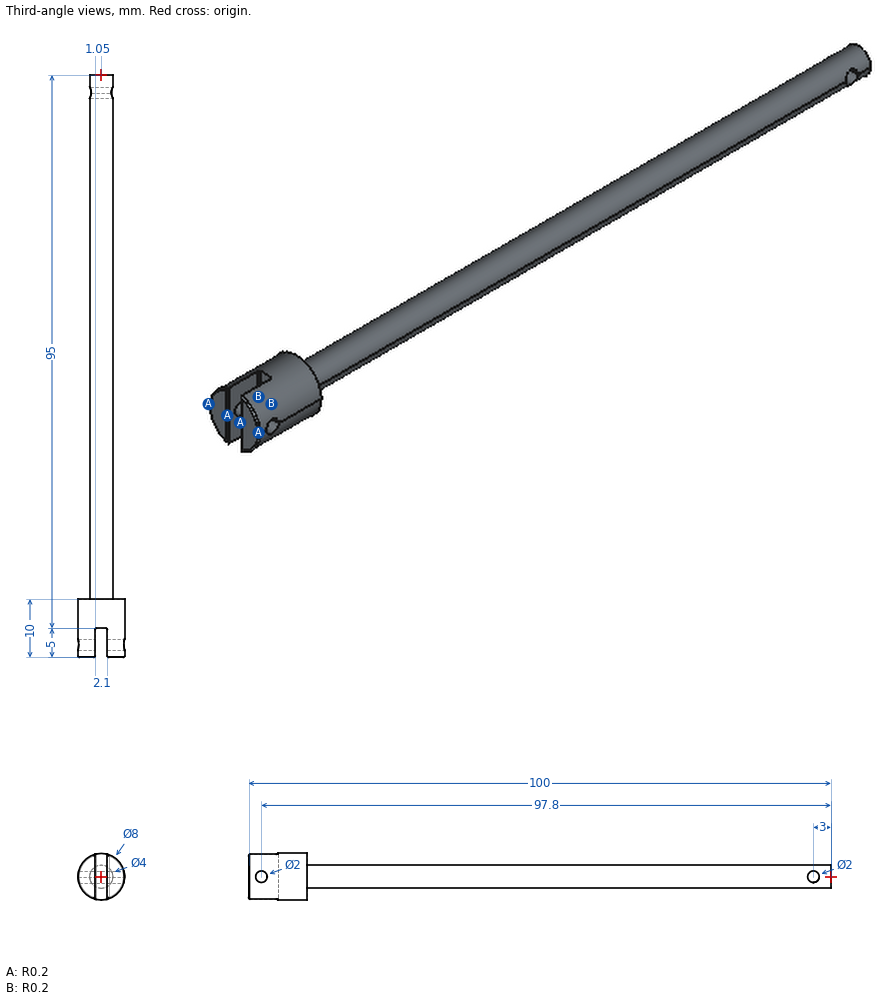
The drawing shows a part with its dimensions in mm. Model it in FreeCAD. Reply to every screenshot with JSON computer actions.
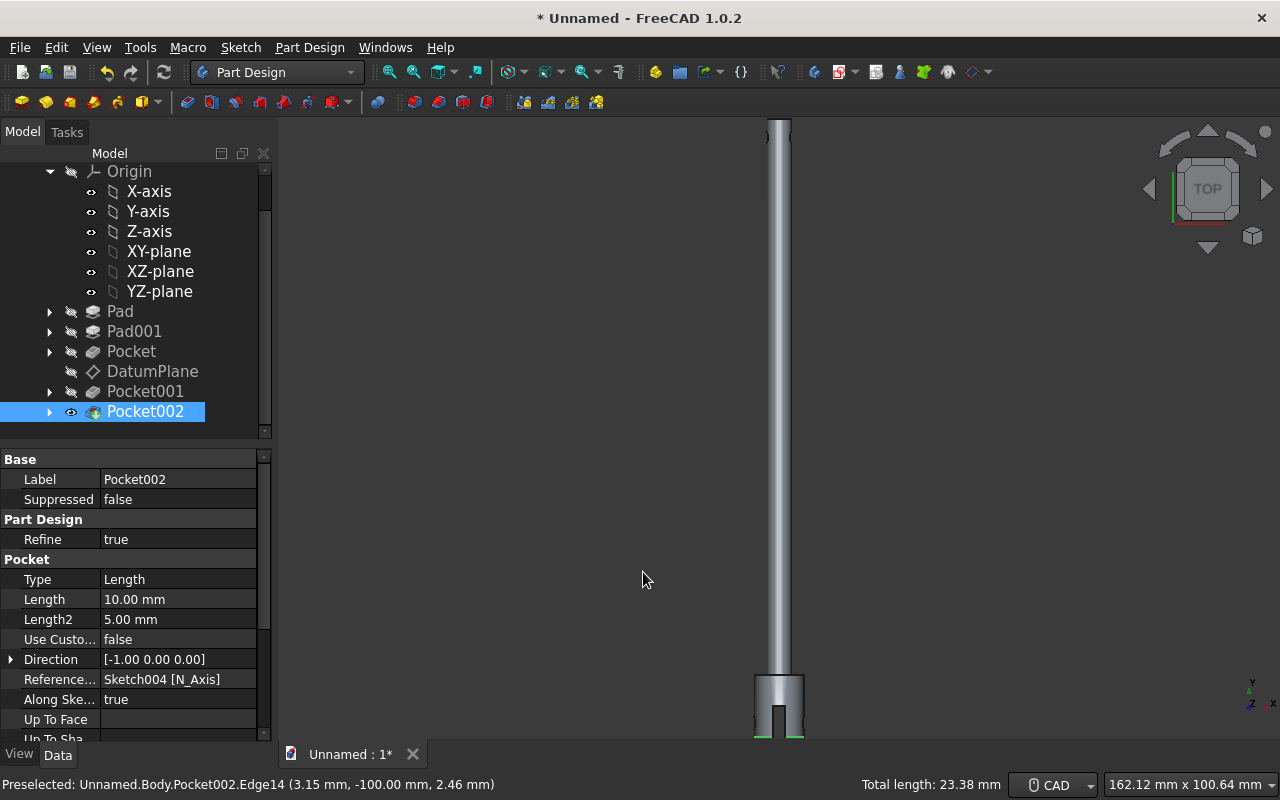
{"action": "key", "text": "1"}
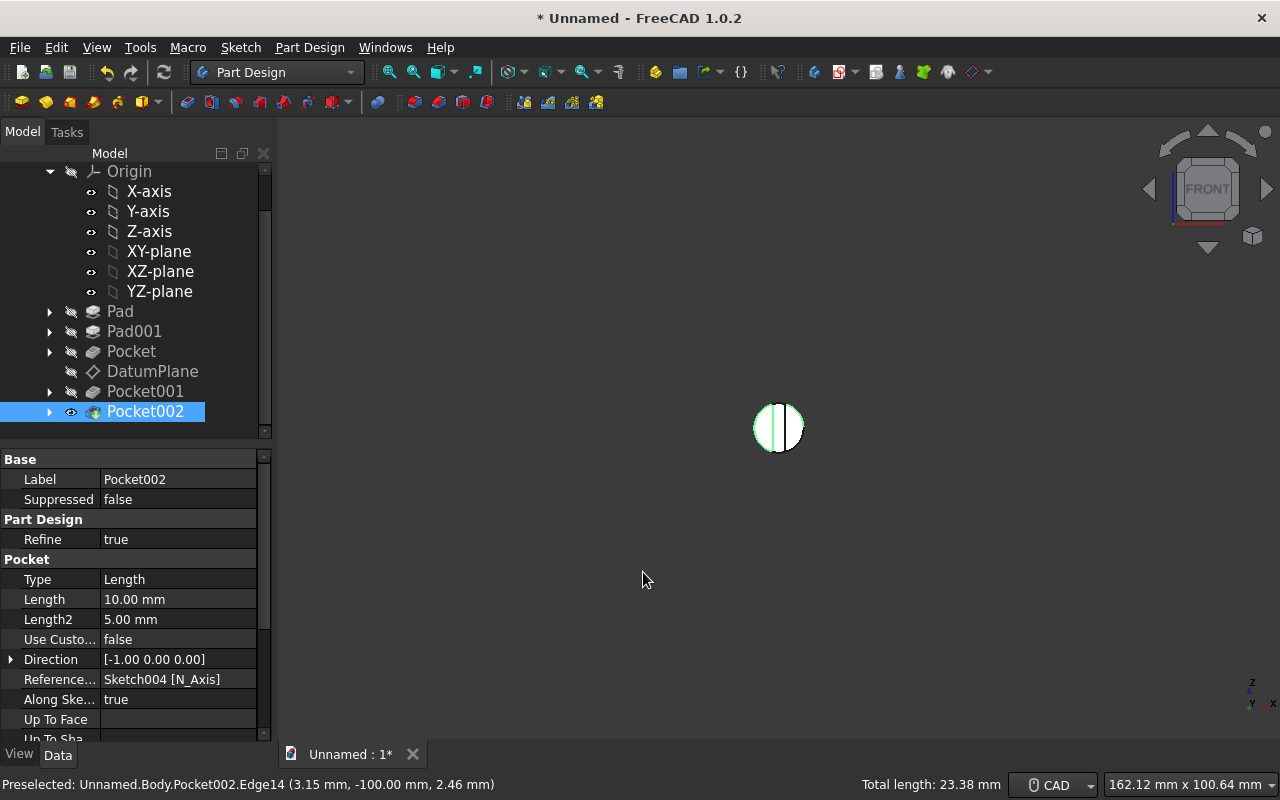
{"action": "left_click", "coordinate": [390, 72]}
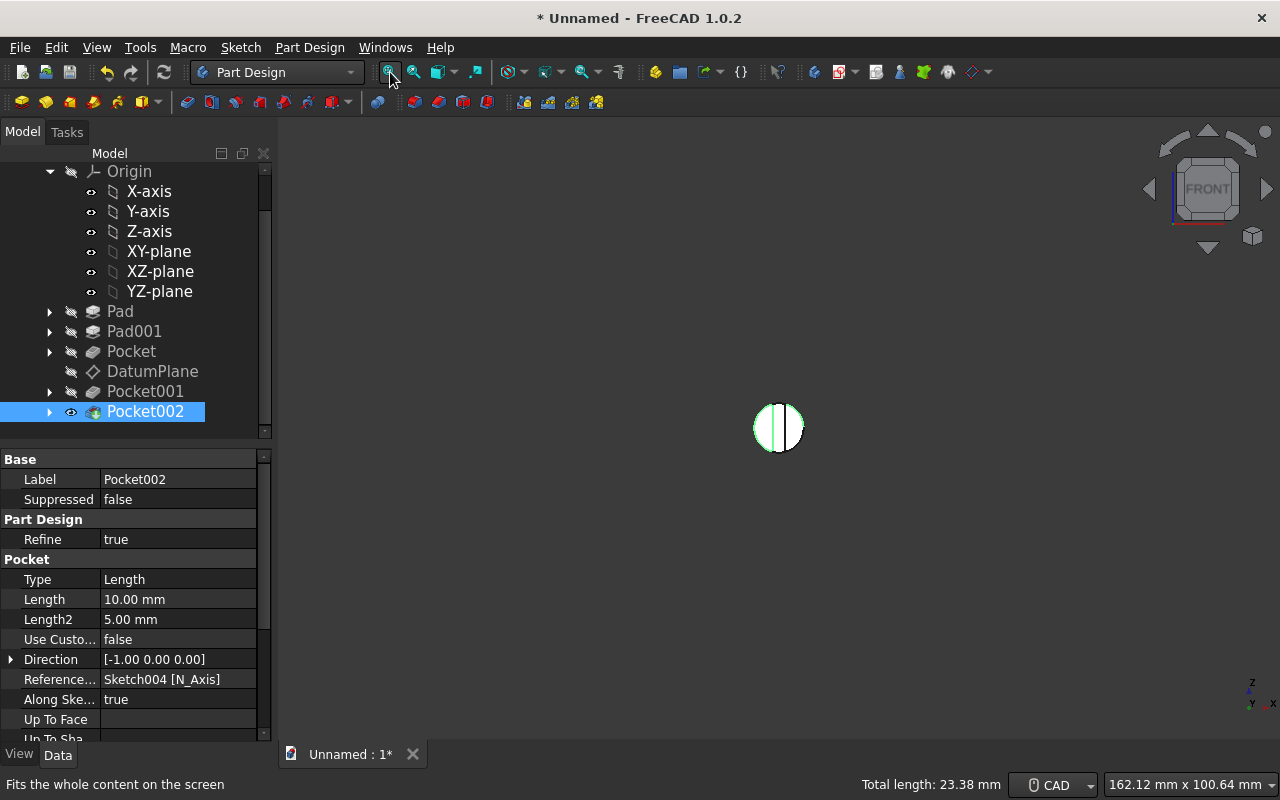
{"action": "left_click", "coordinate": [785, 427], "text": "ctrl"}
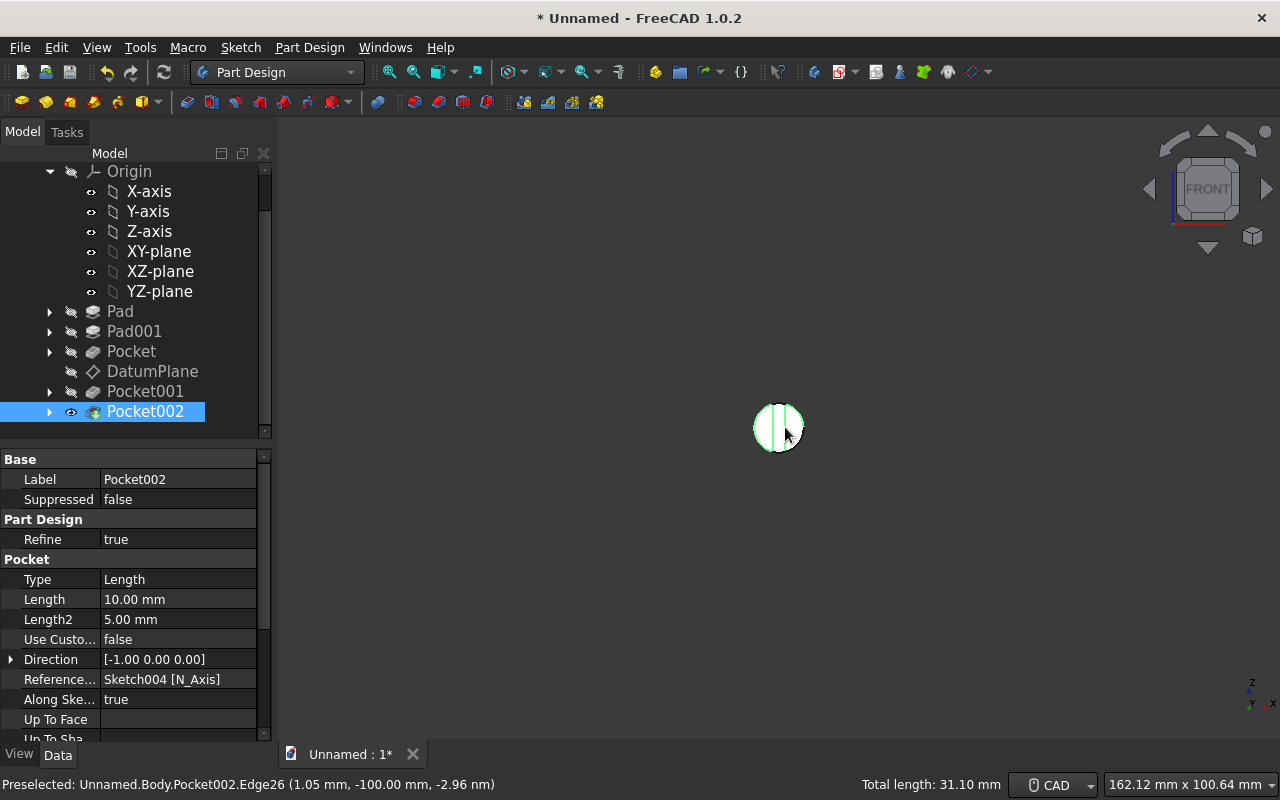
{"action": "left_click", "coordinate": [416, 102]}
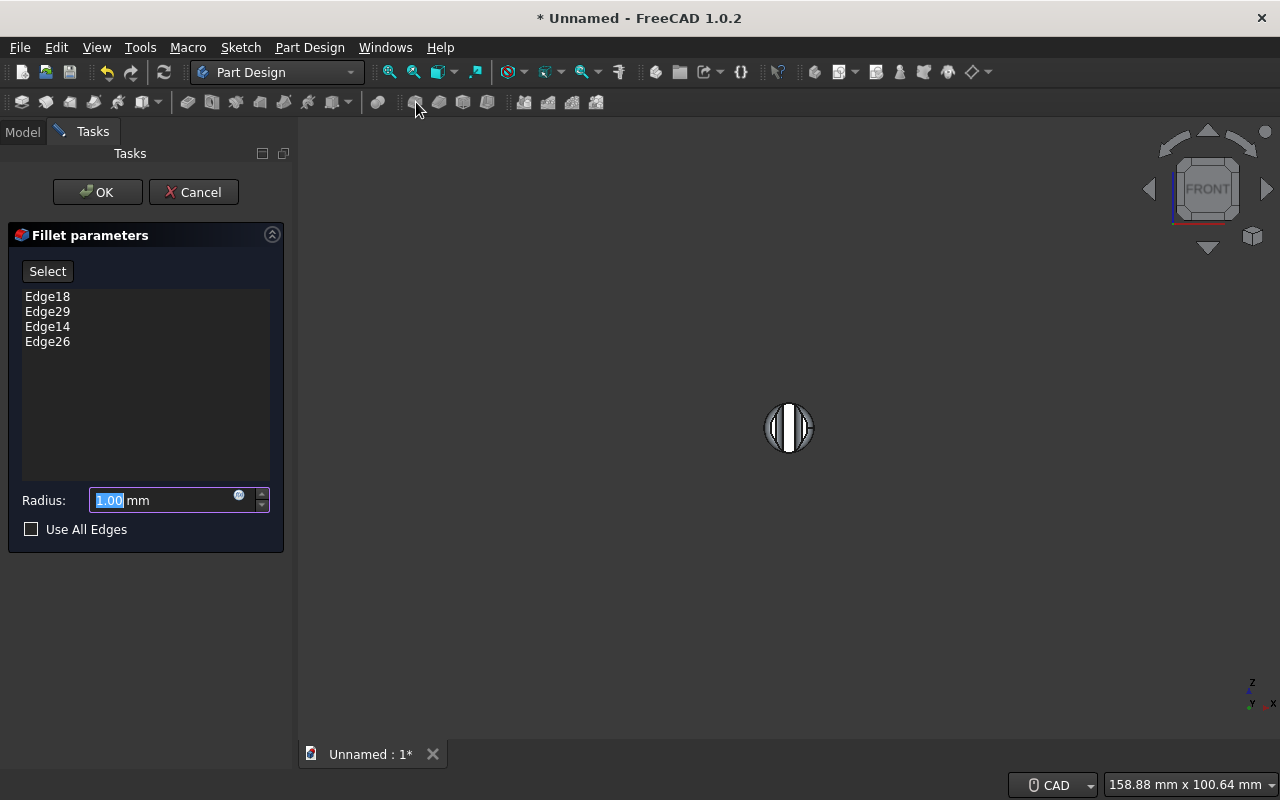
{"action": "type", "text": "0.2"}
{"action": "key", "text": "Tab"}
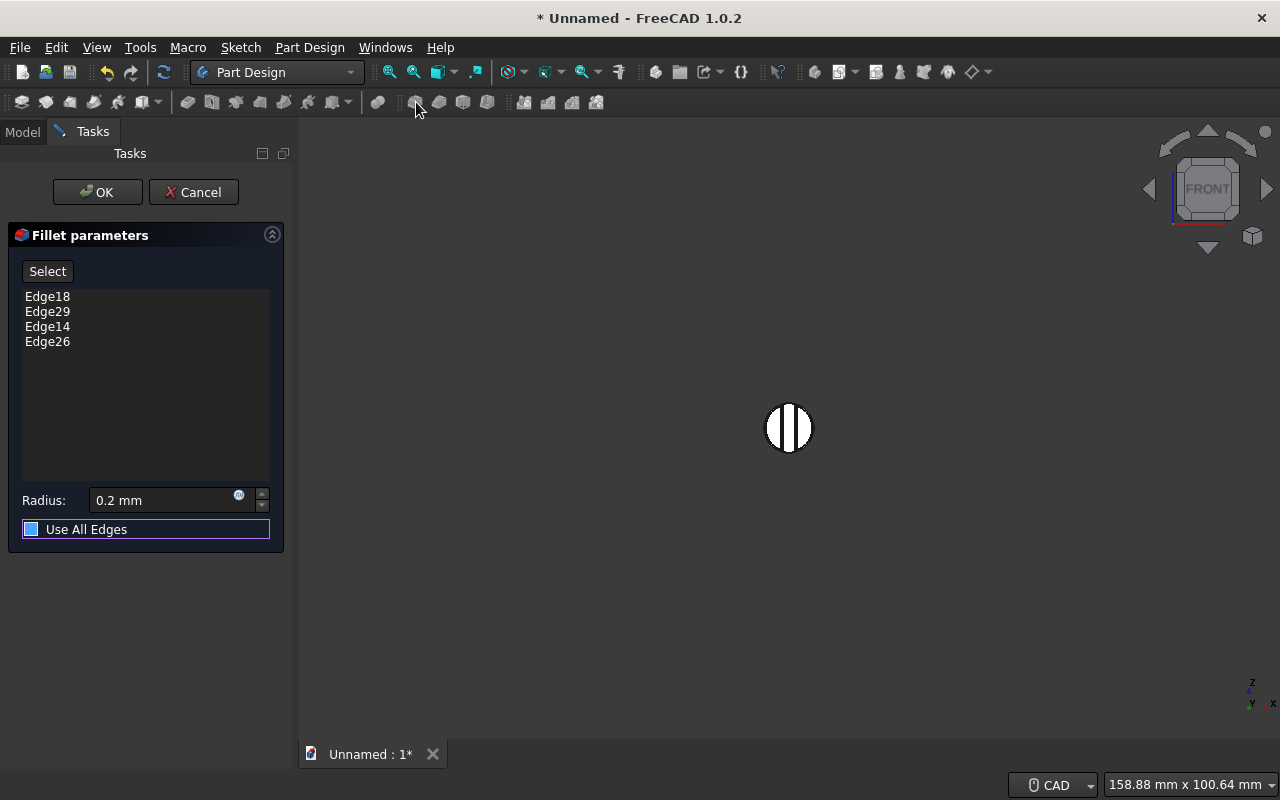
{"action": "left_click", "coordinate": [98, 192]}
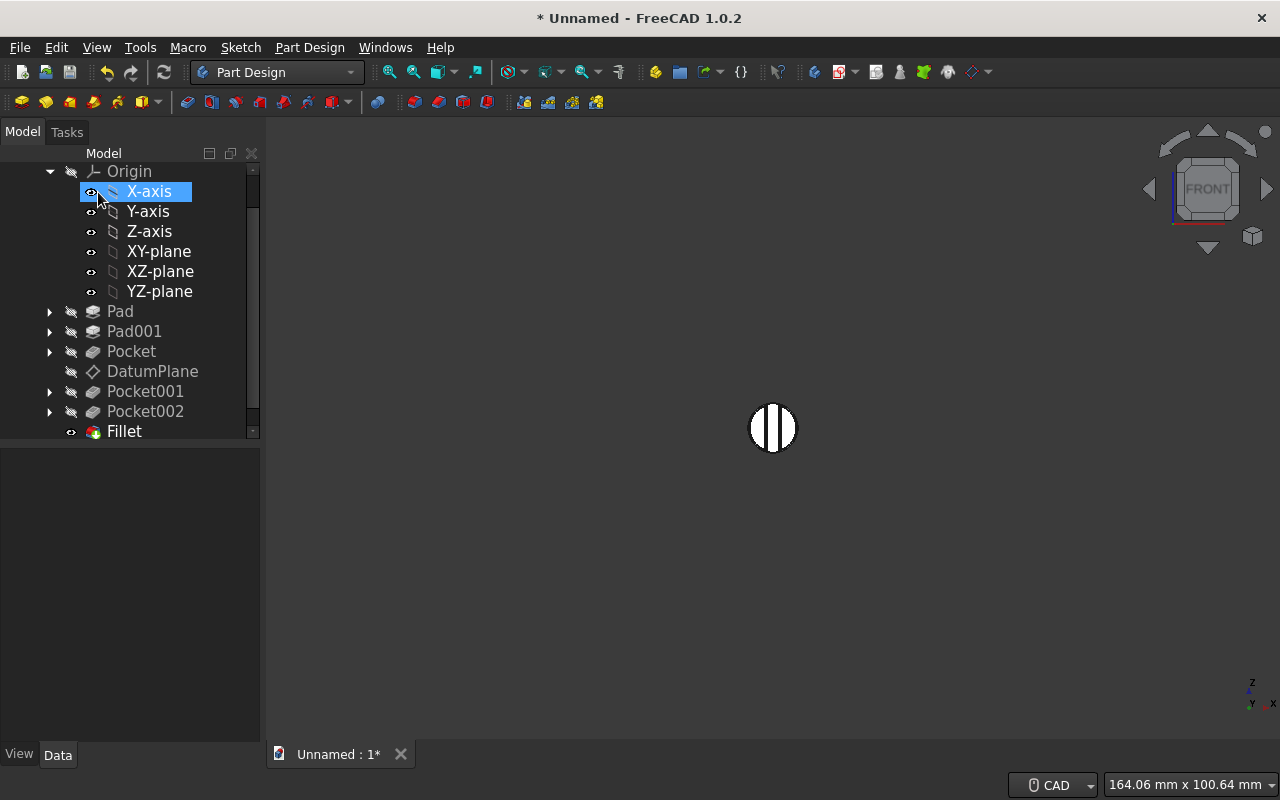
{"action": "left_click", "coordinate": [390, 72]}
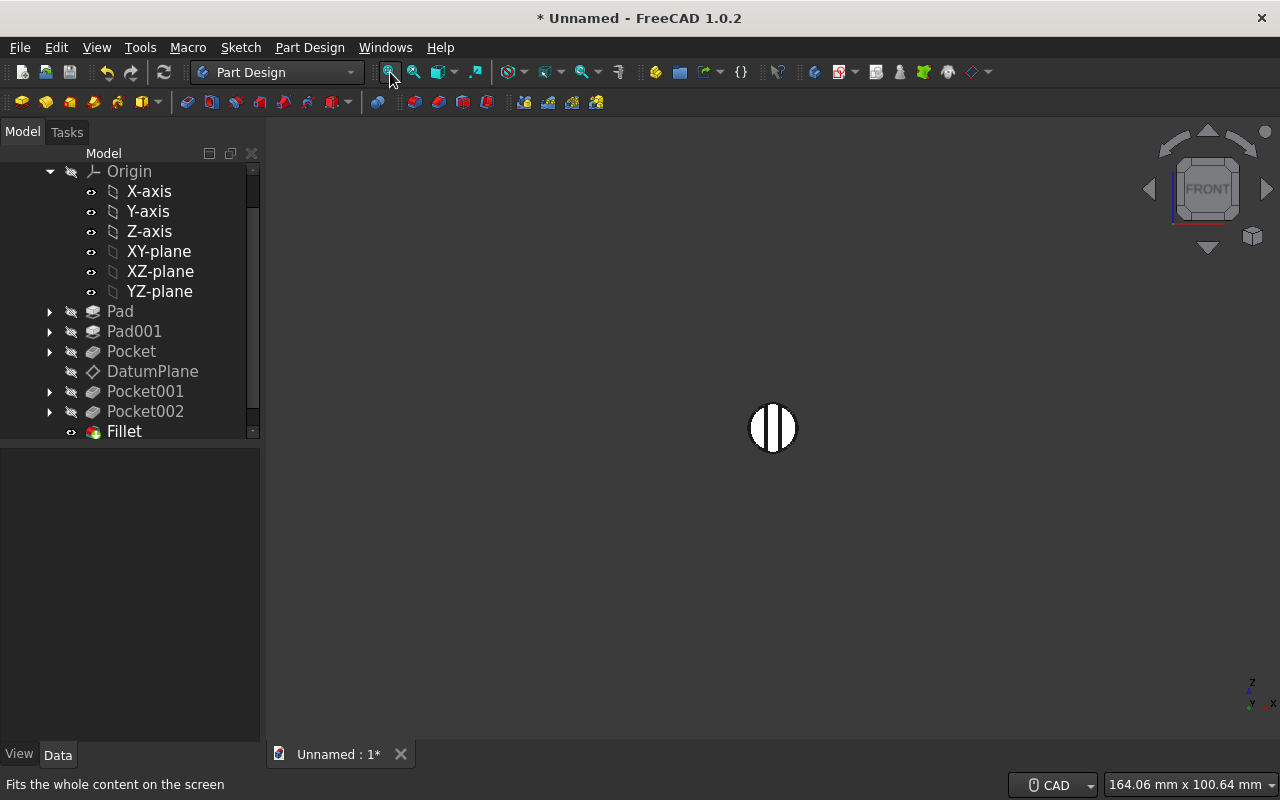
{"action": "key", "text": "0"}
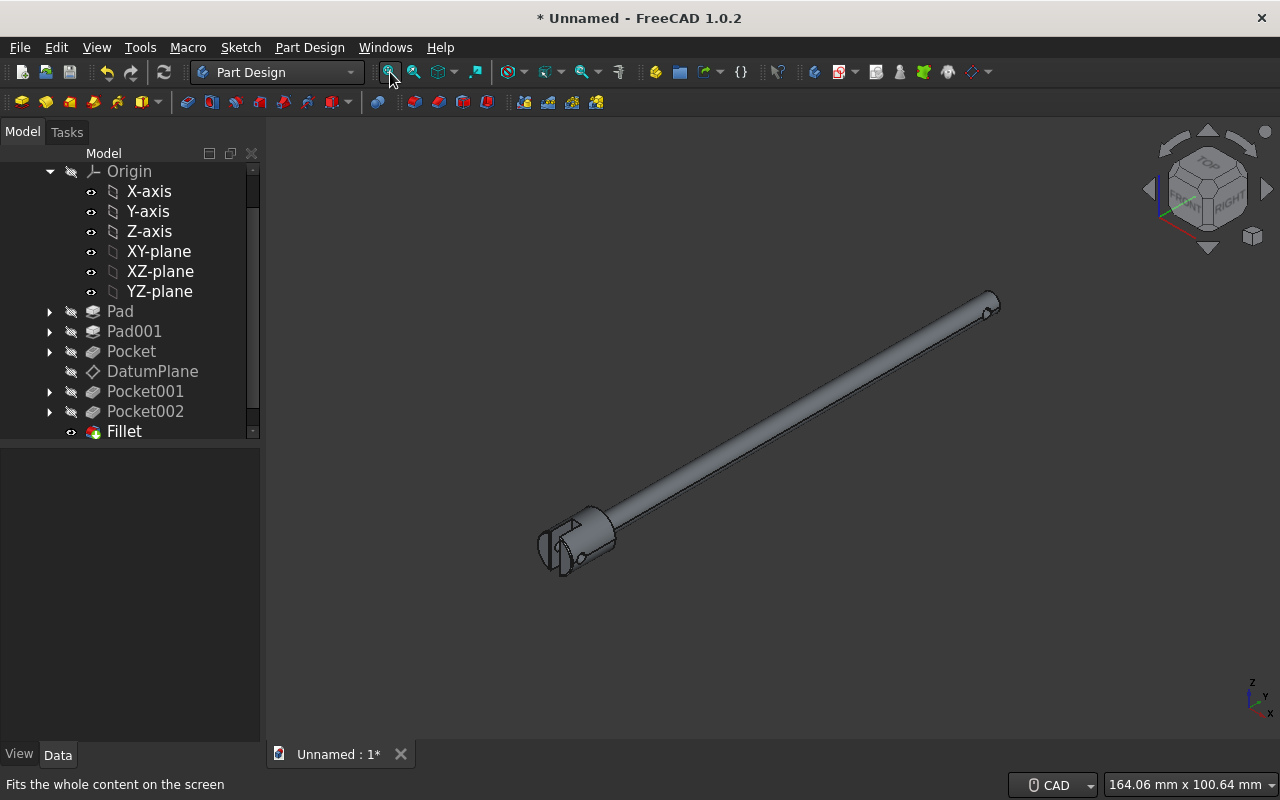
{"action": "key", "text": "2"}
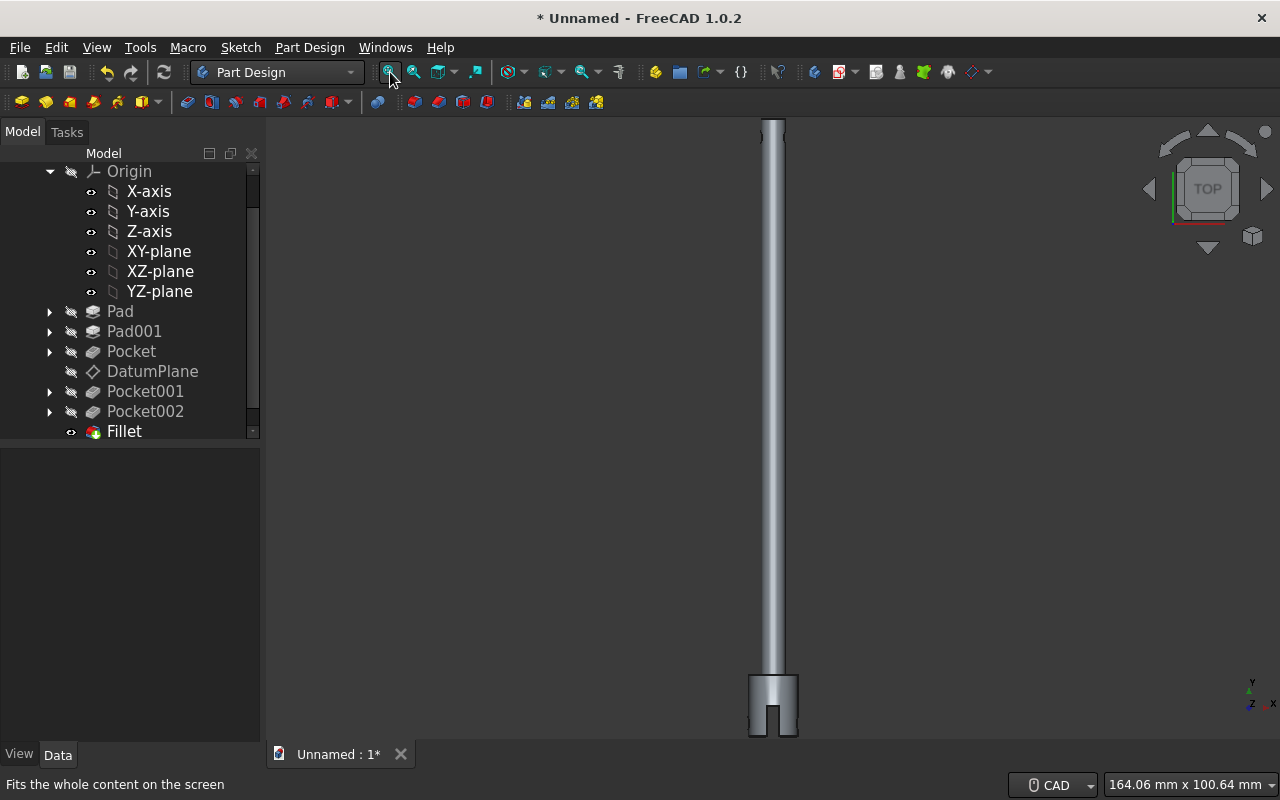
{"action": "key", "text": "1"}